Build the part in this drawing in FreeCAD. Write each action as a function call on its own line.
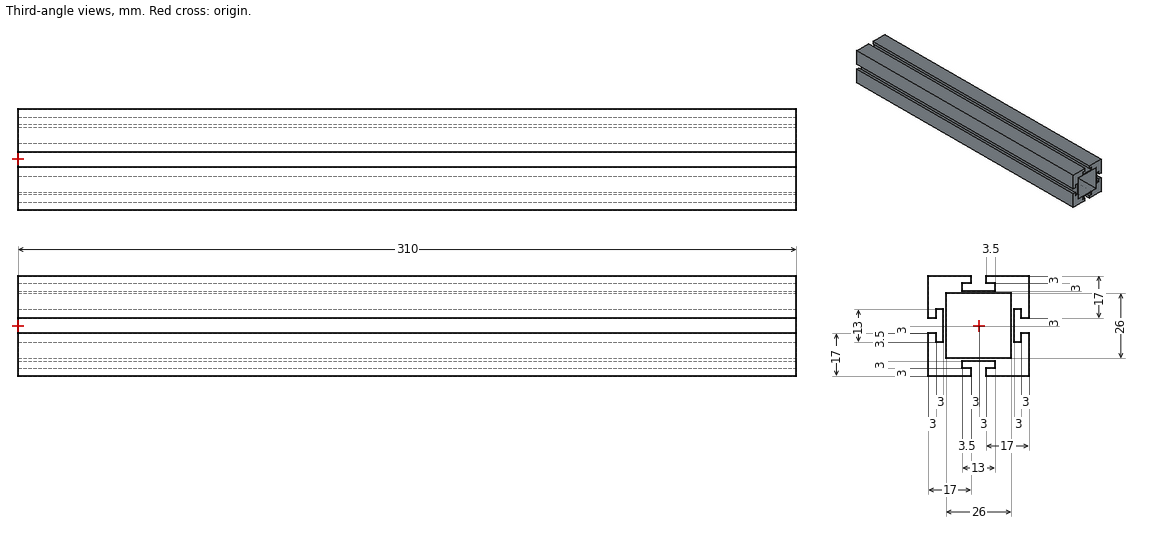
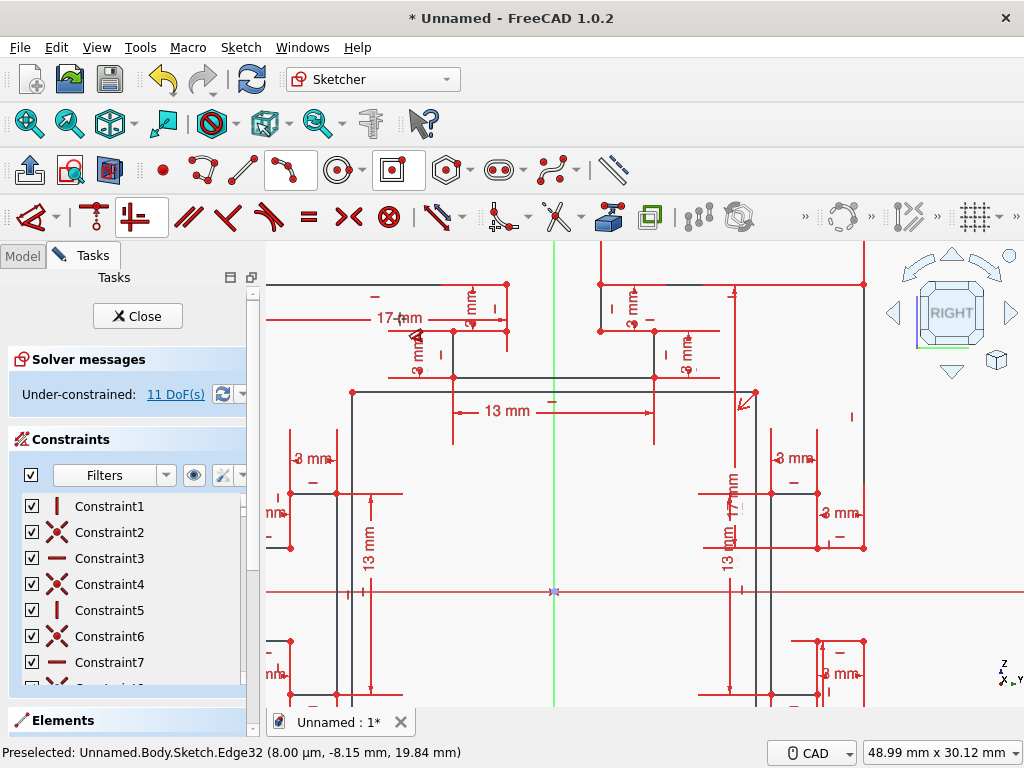
scroll(595, 378, down, 4)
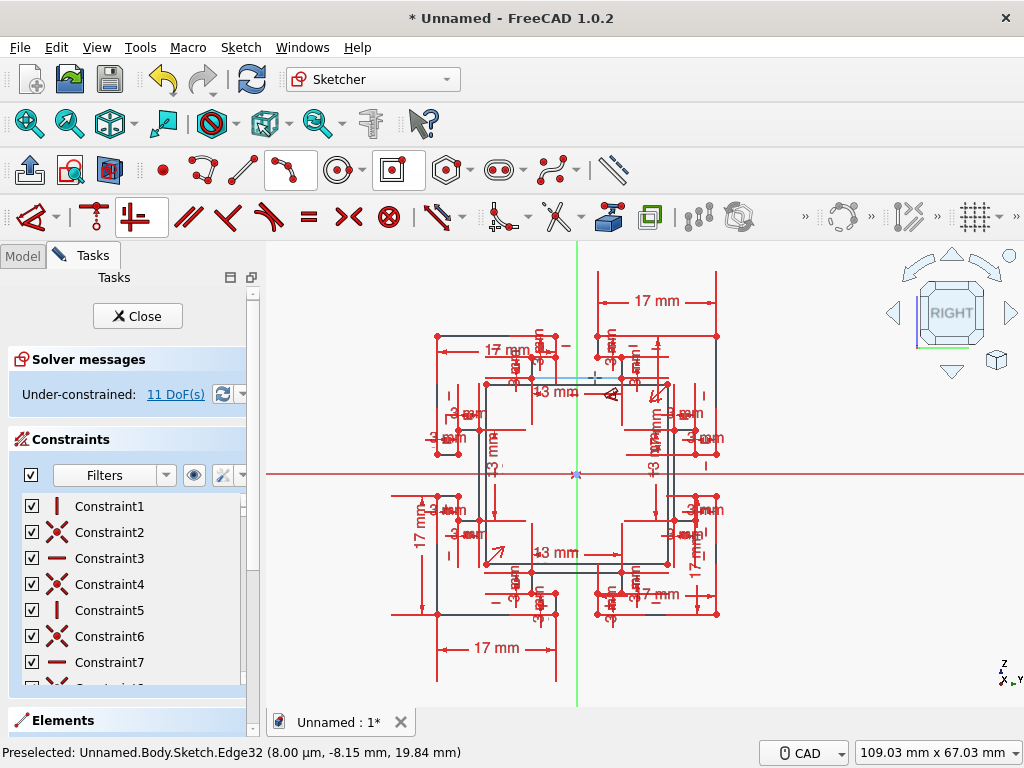
click(437, 372)
click(403, 368)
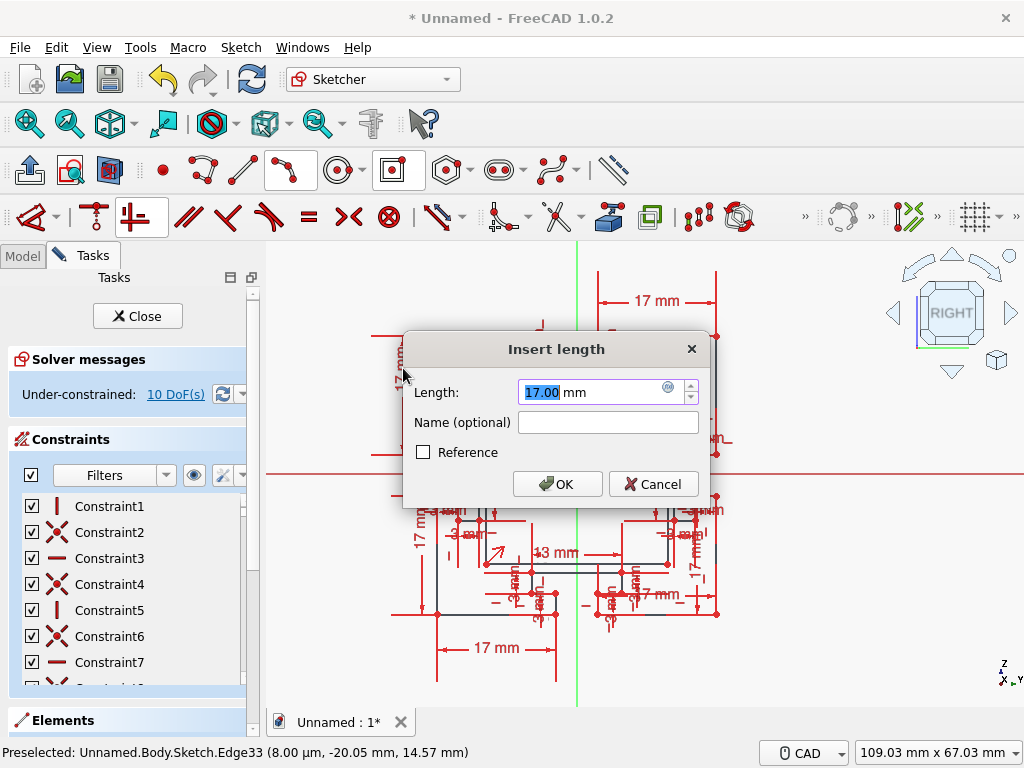
text(17)
key(Return)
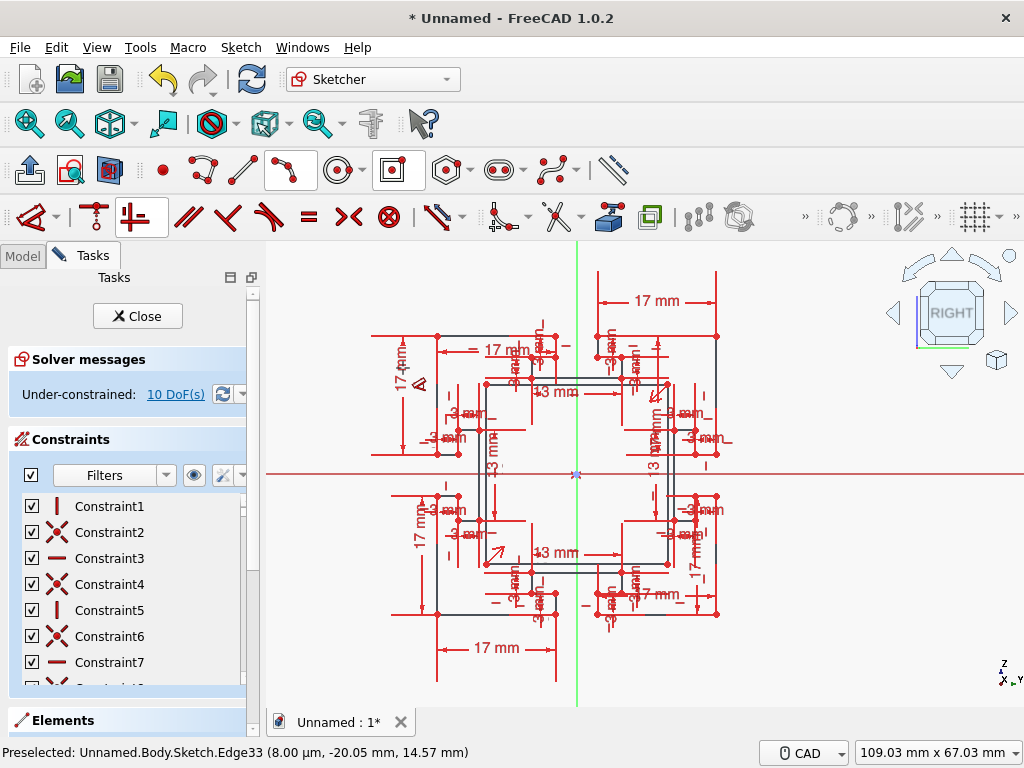
click(522, 564)
click(535, 506)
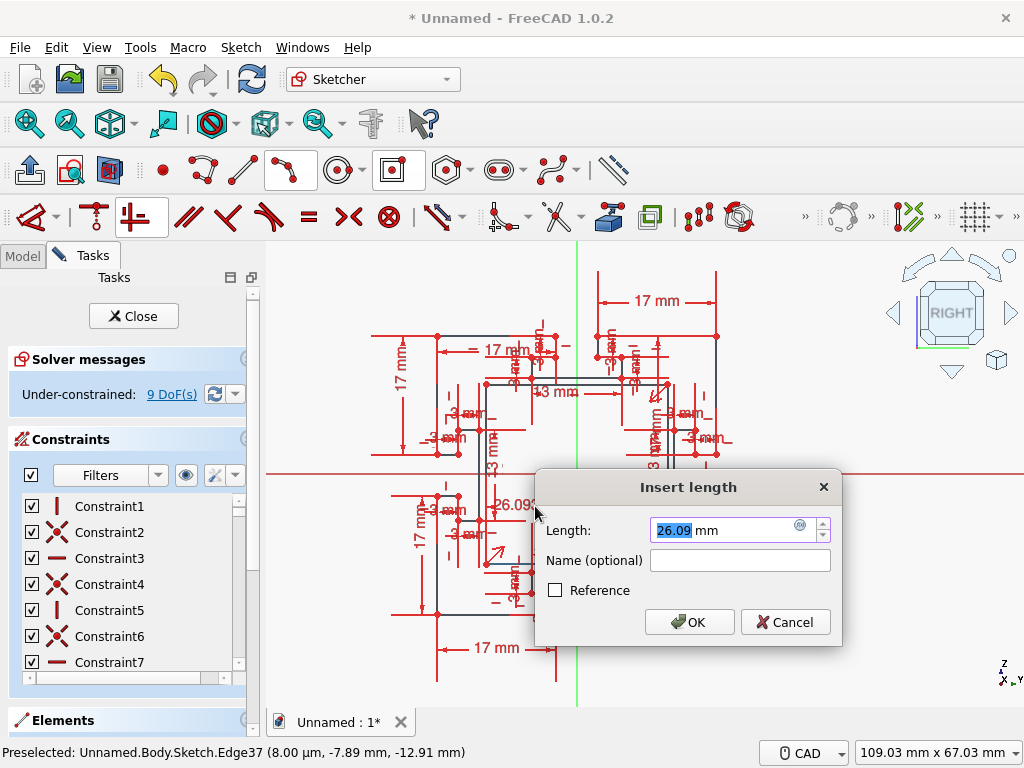
text(26)
key(Return)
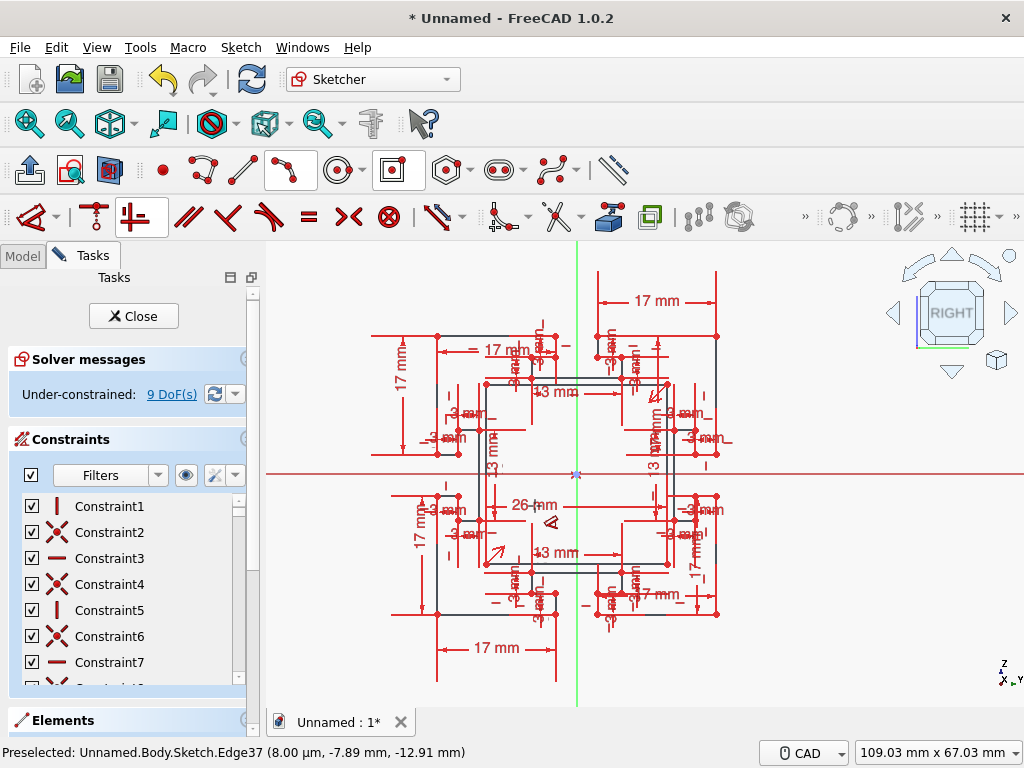
scroll(667, 528, up, 2)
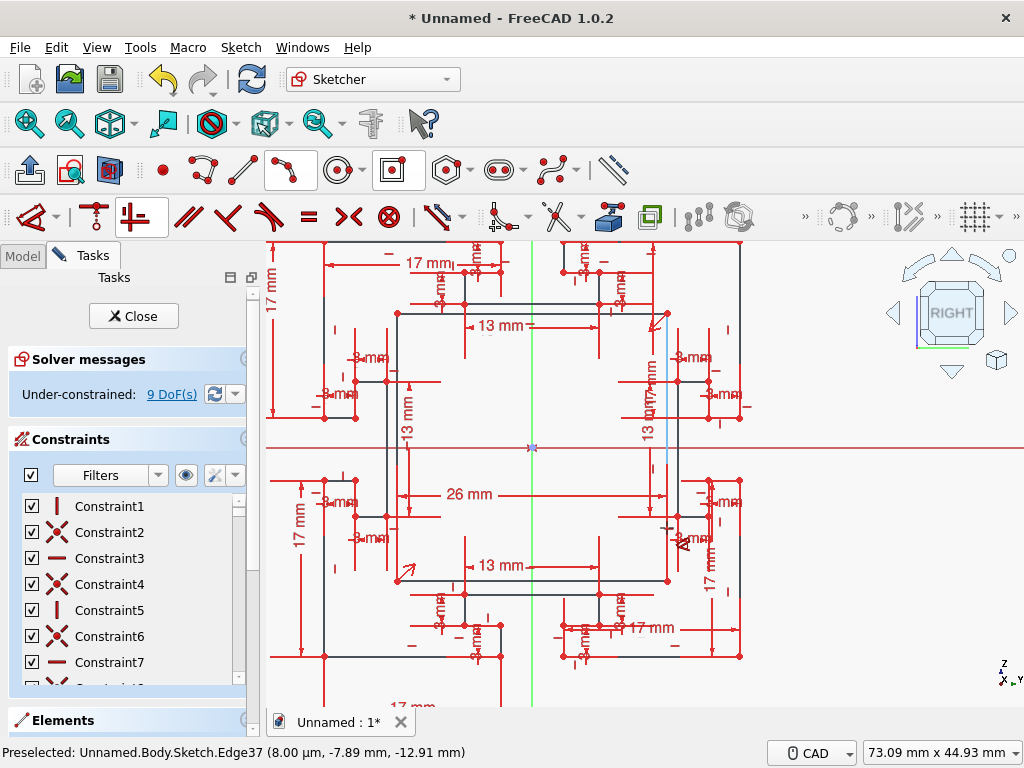
click(667, 528)
click(633, 509)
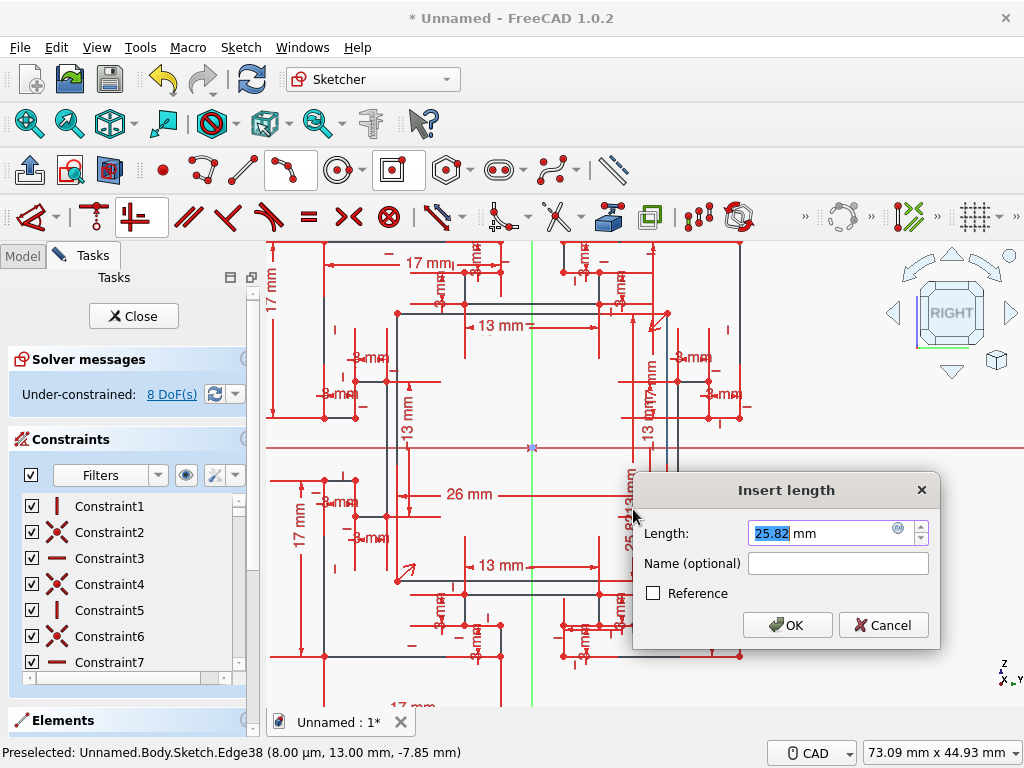
text(26)
key(Return)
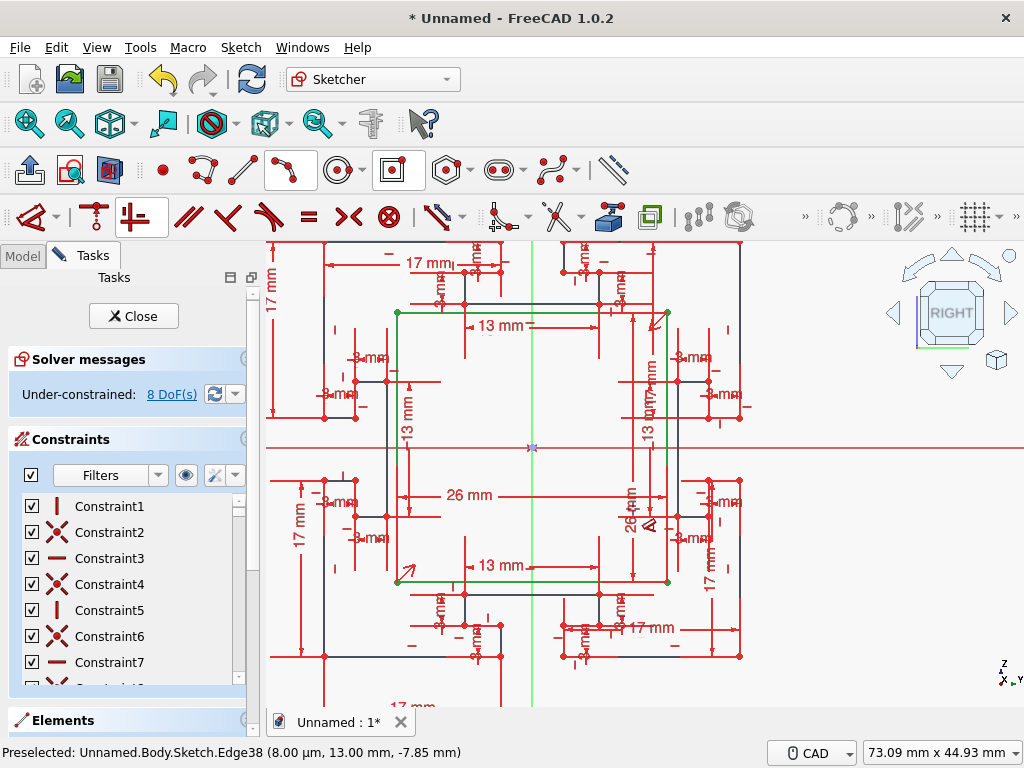
scroll(355, 481, up, 2)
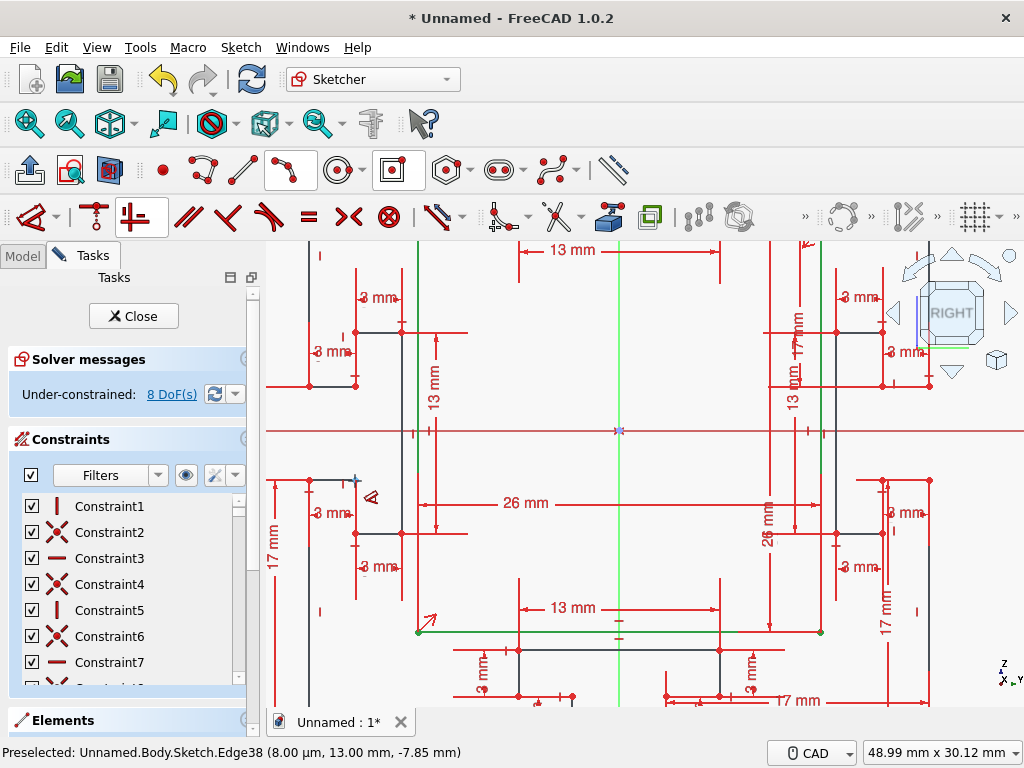
click(356, 480)
click(322, 455)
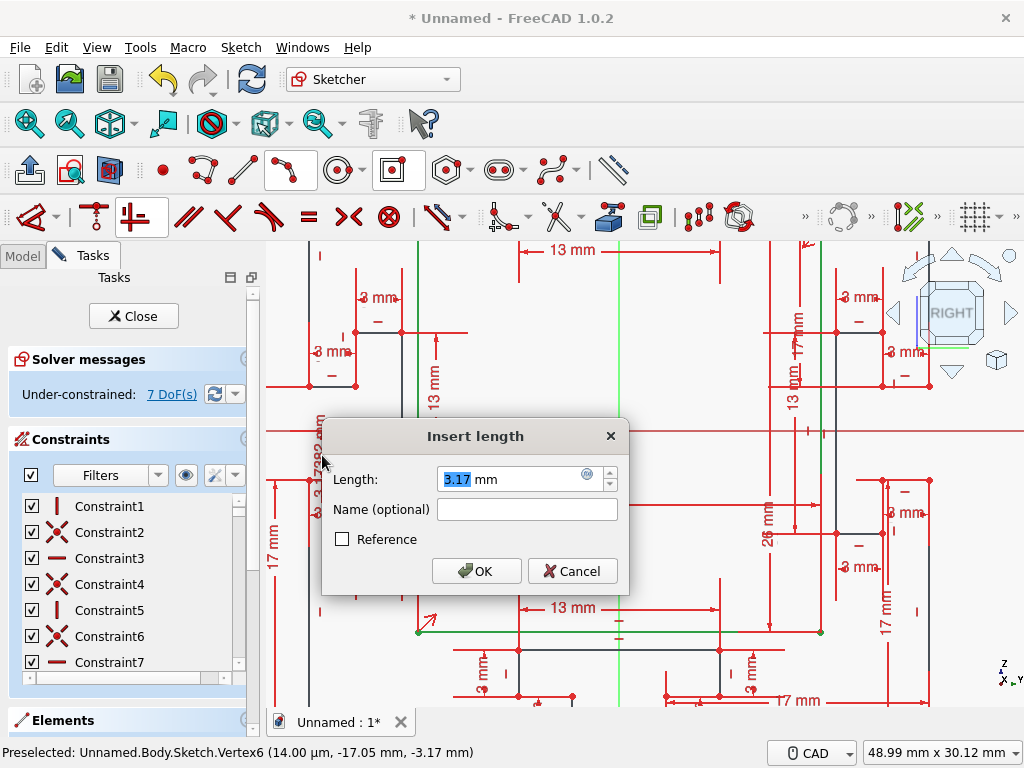
text(3)
key(Return)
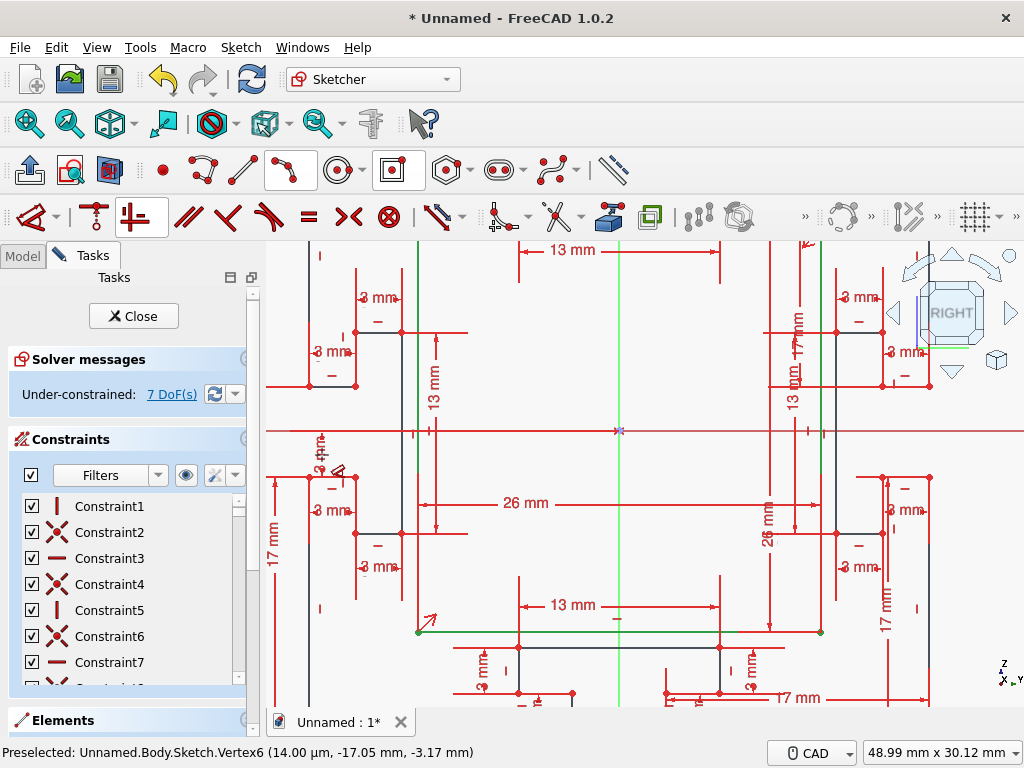
scroll(542, 509, down, 4)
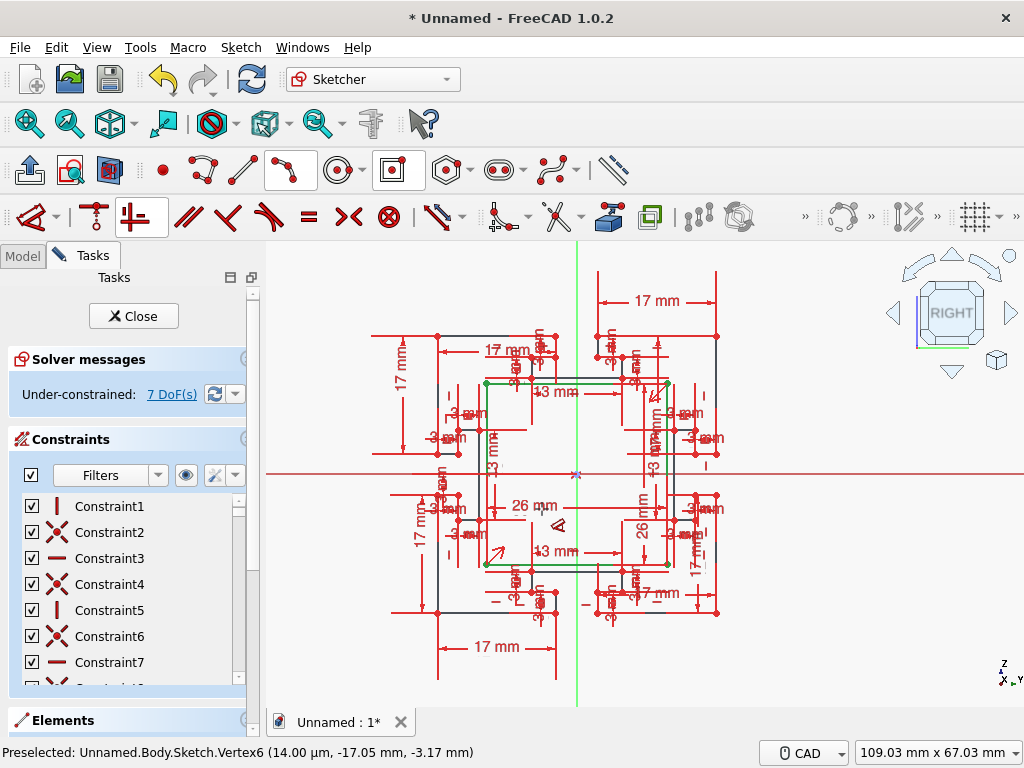
scroll(556, 613, up, 4)